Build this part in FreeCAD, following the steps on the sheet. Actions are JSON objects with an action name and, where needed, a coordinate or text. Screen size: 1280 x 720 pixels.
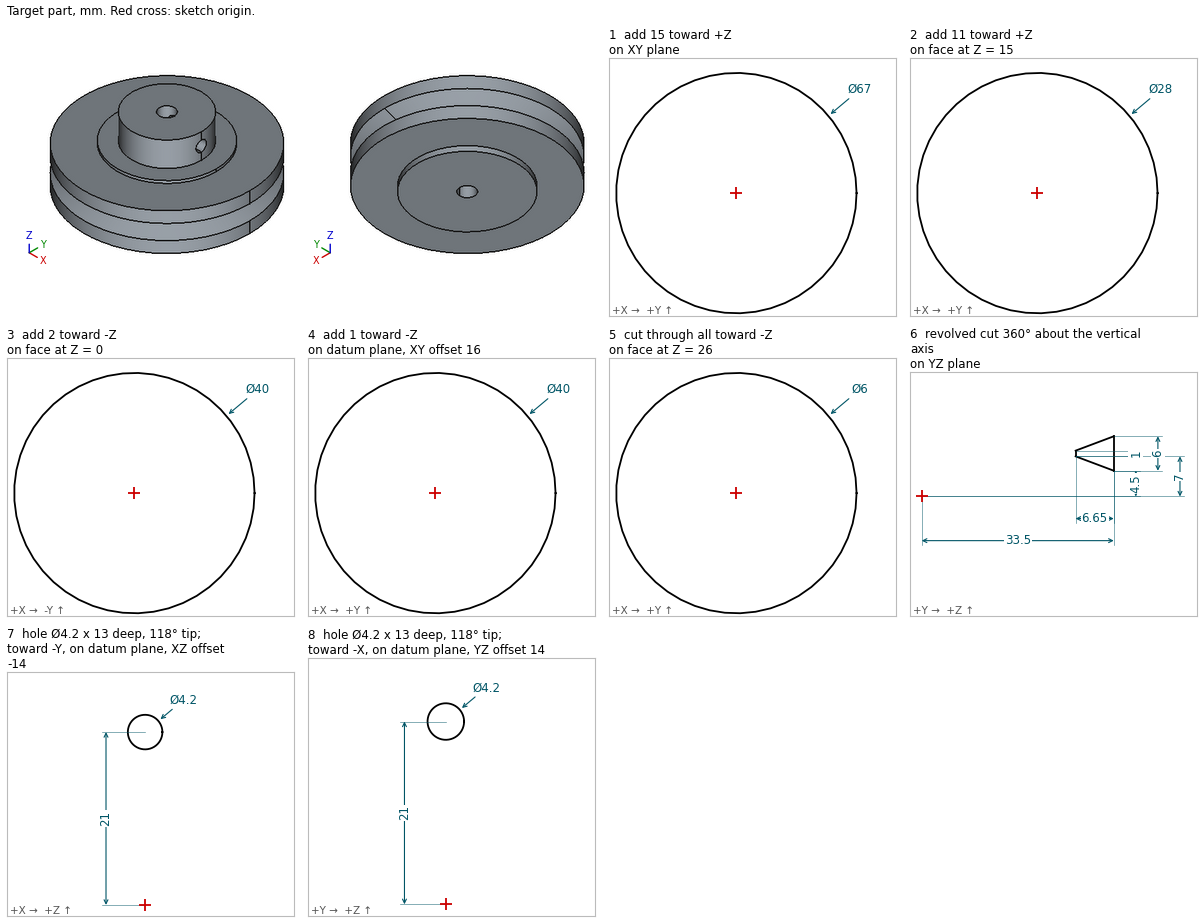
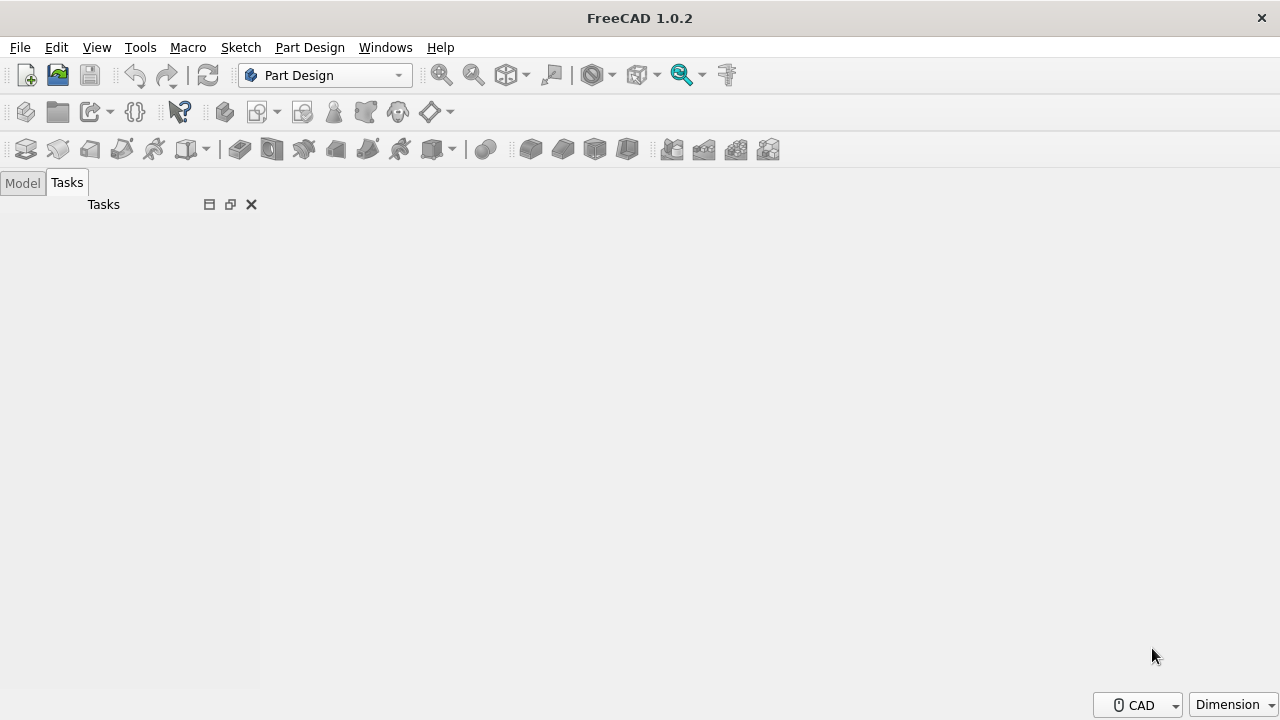
{"action": "left_click", "coordinate": [26, 76]}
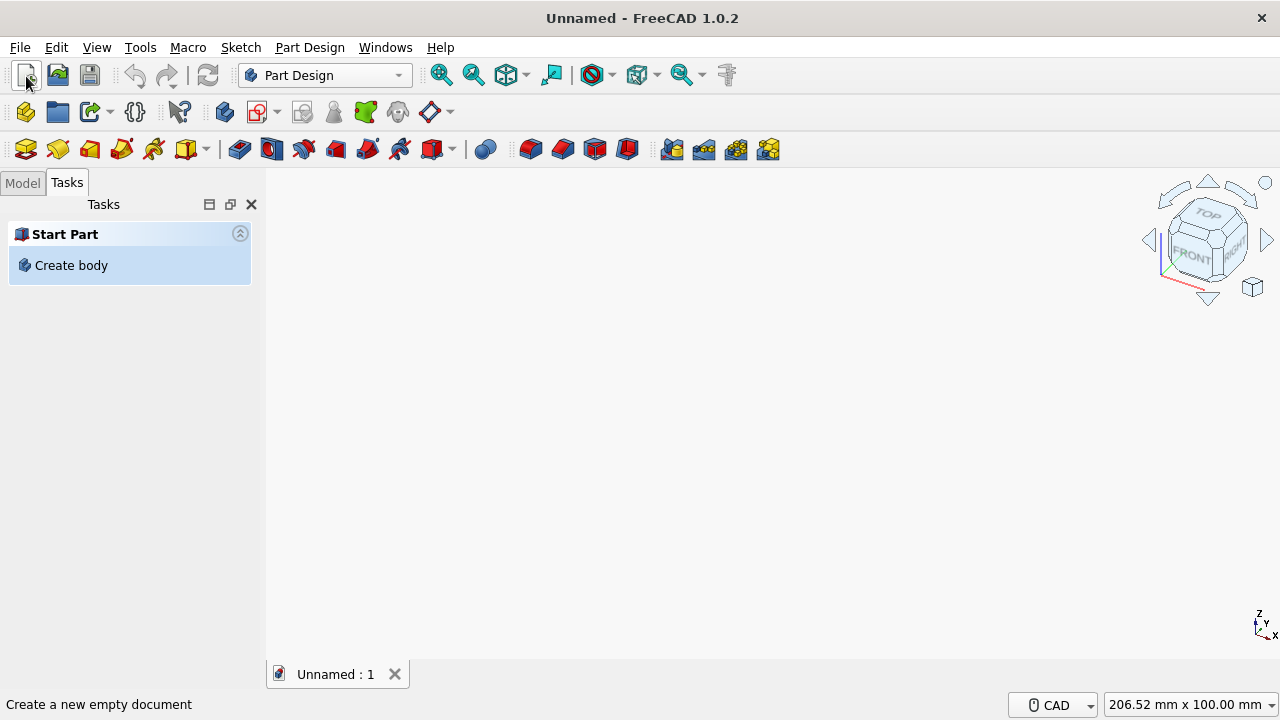
{"action": "left_click", "coordinate": [258, 112]}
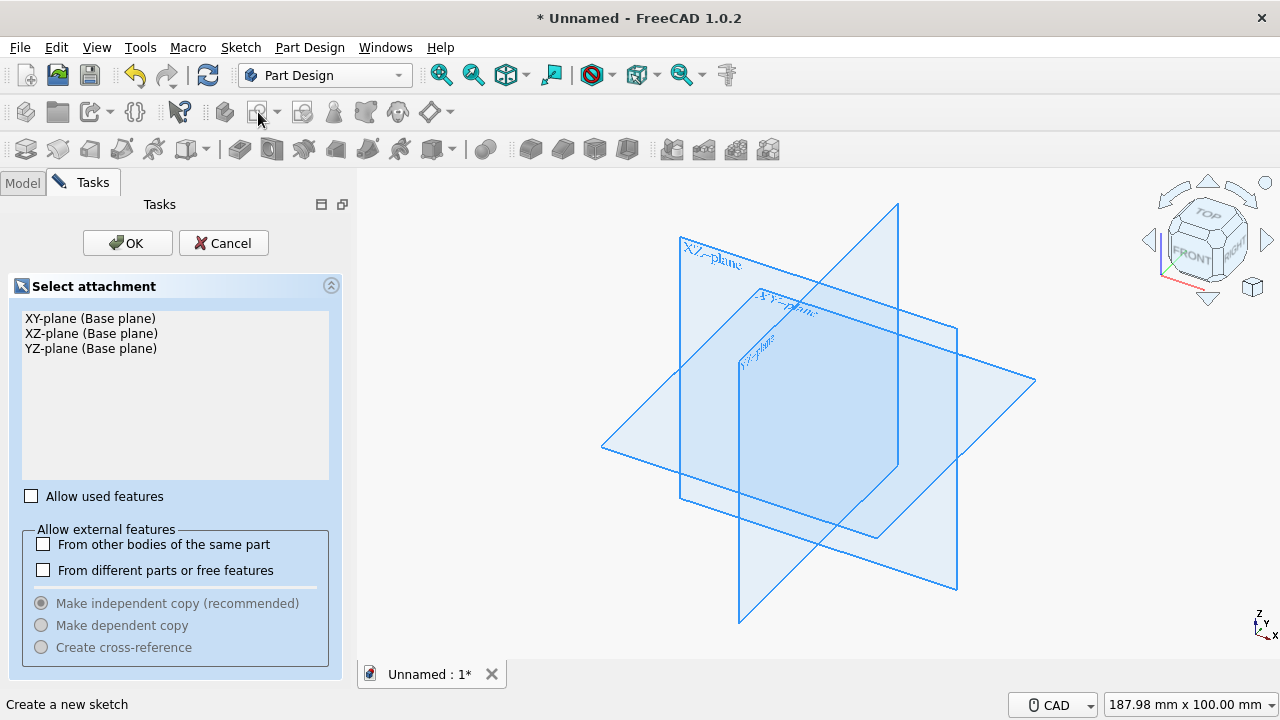
{"action": "left_click", "coordinate": [82, 318]}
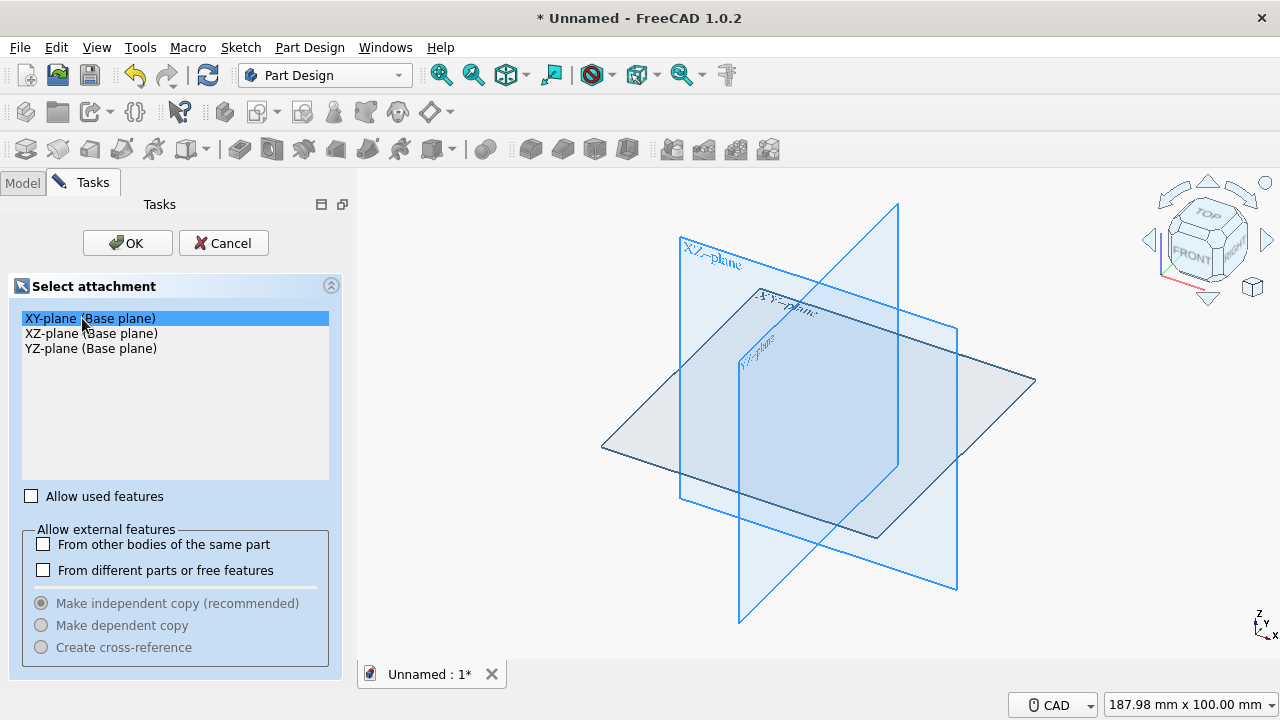
{"action": "left_click", "coordinate": [128, 243]}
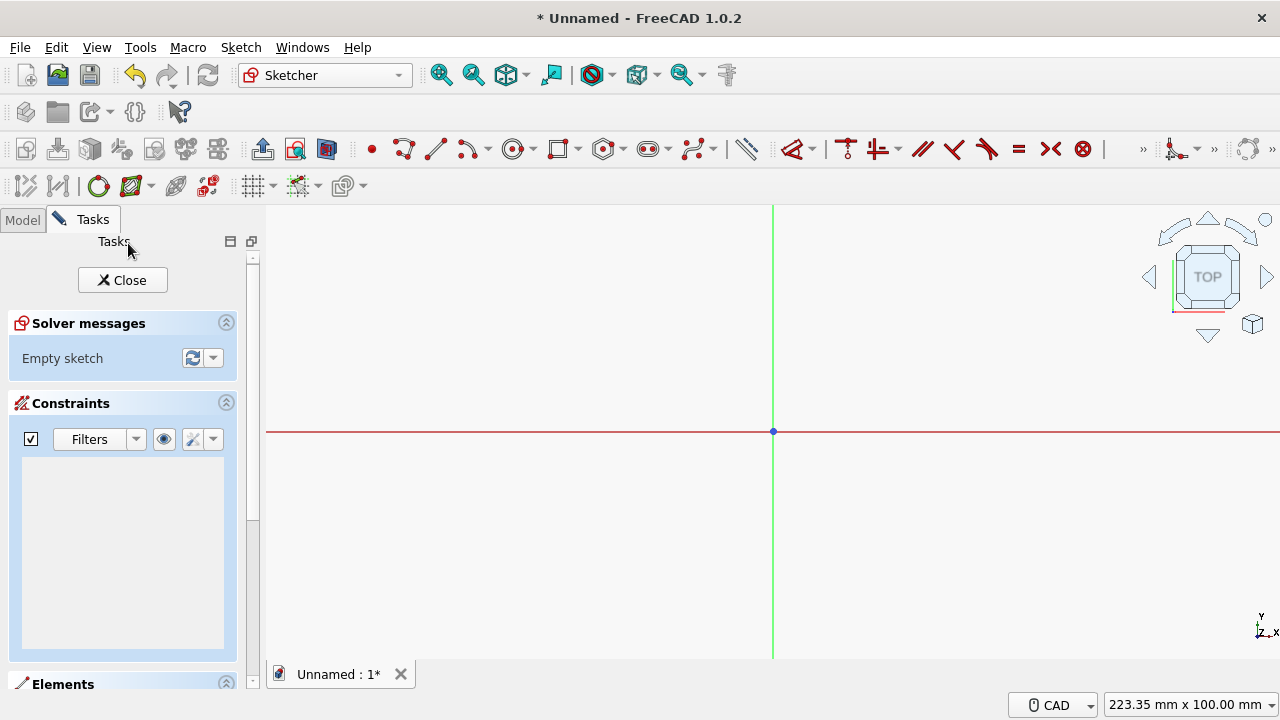
{"action": "left_click", "coordinate": [514, 150]}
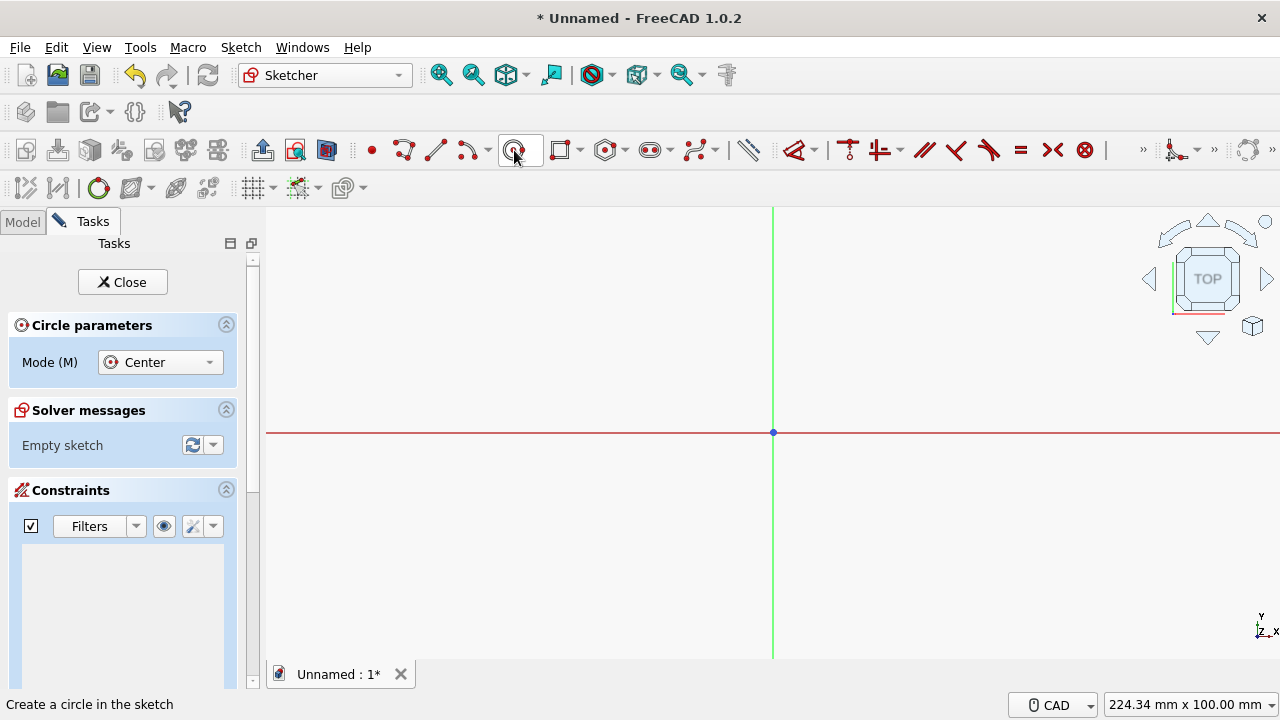
{"action": "left_click", "coordinate": [773, 433]}
{"action": "left_click", "coordinate": [880, 326]}
{"action": "key", "text": "Escape"}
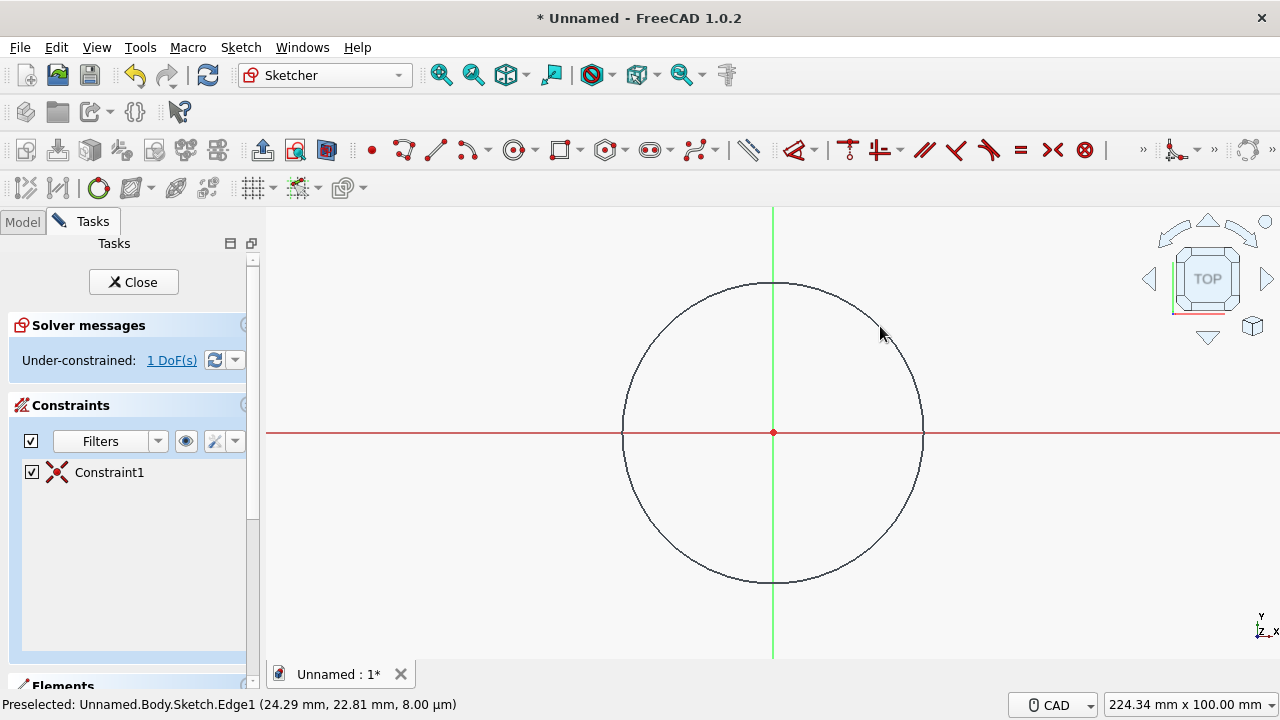
{"action": "left_click", "coordinate": [879, 326]}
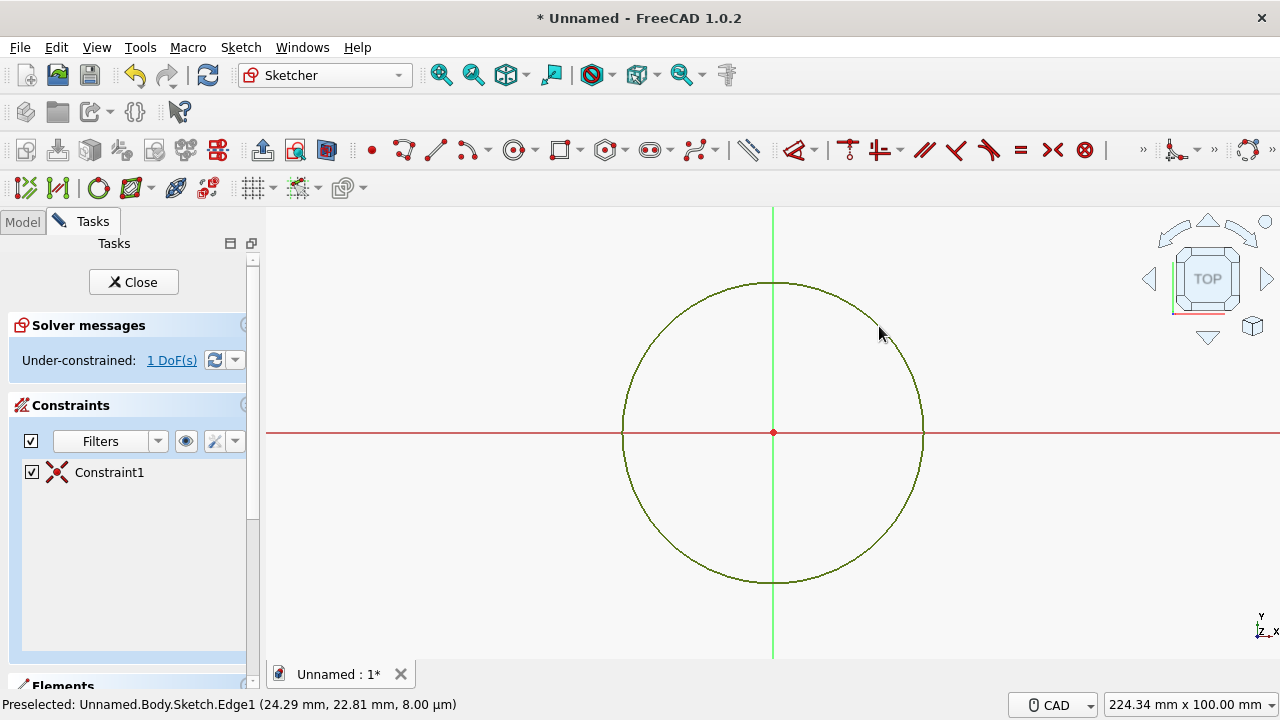
{"action": "key", "text": "k o"}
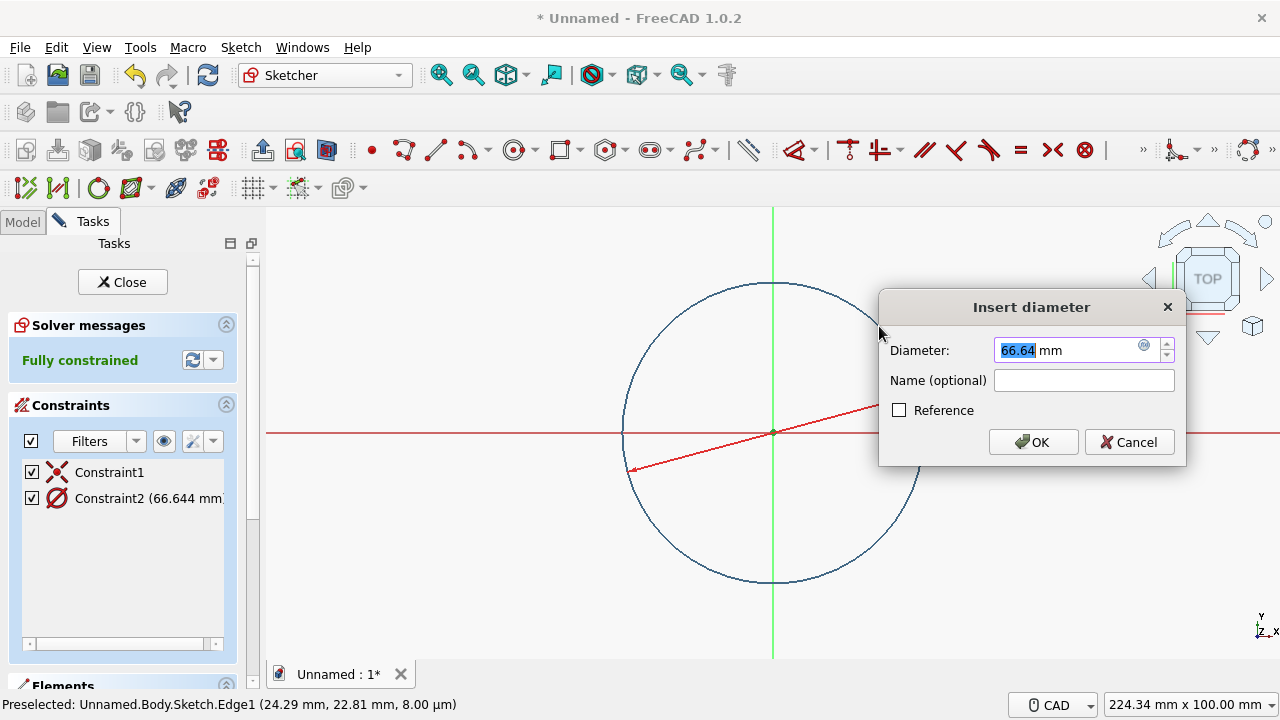
{"action": "type", "text": "67"}
{"action": "key", "text": "Return"}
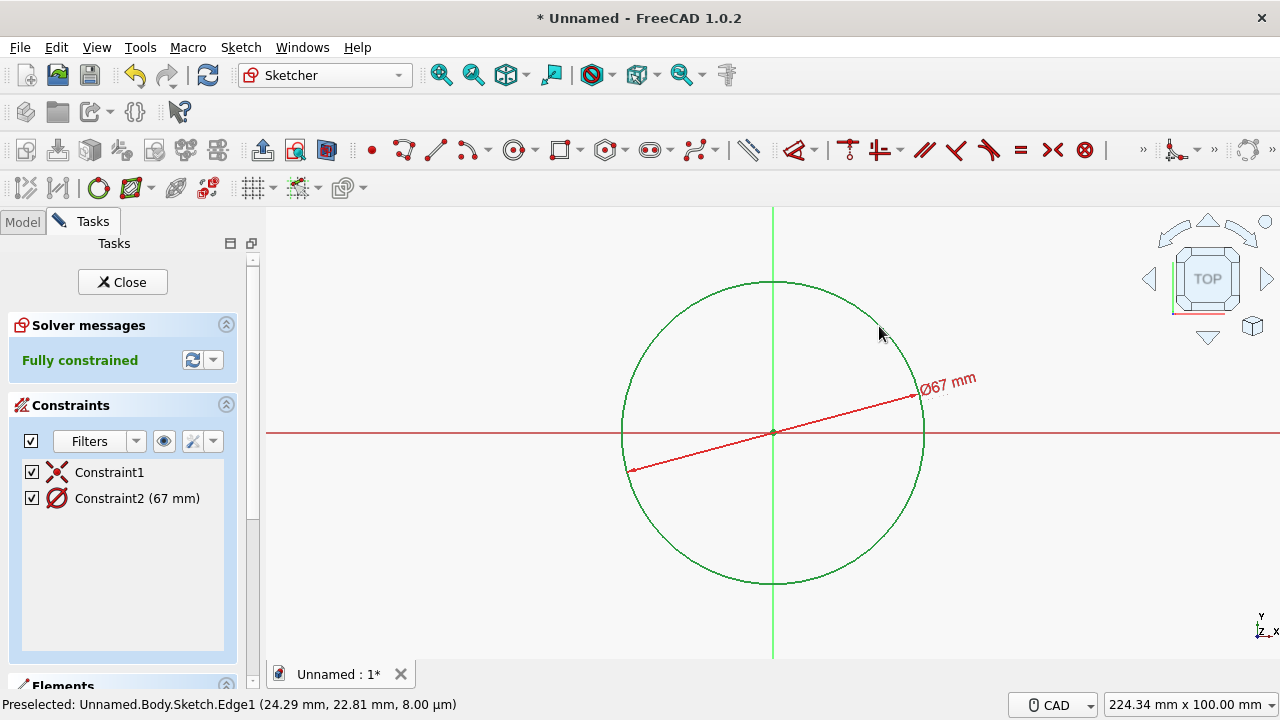
{"action": "left_click", "coordinate": [123, 282]}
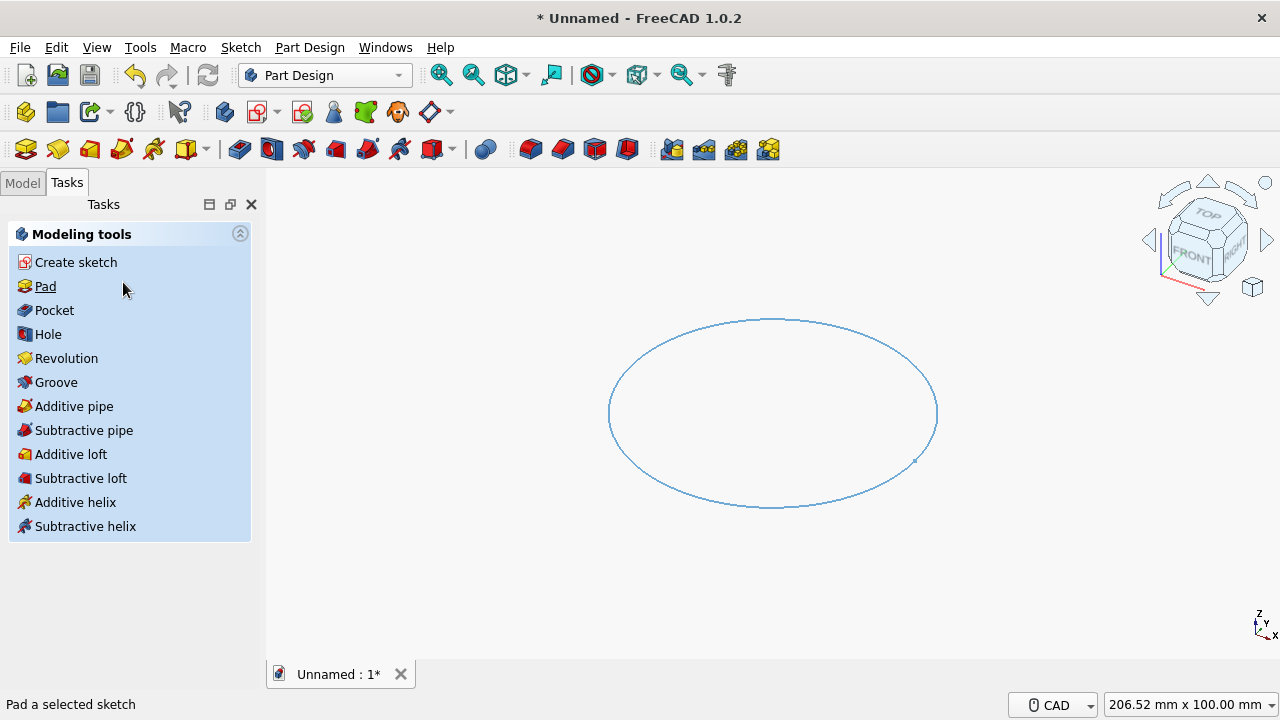
{"action": "left_click", "coordinate": [26, 150]}